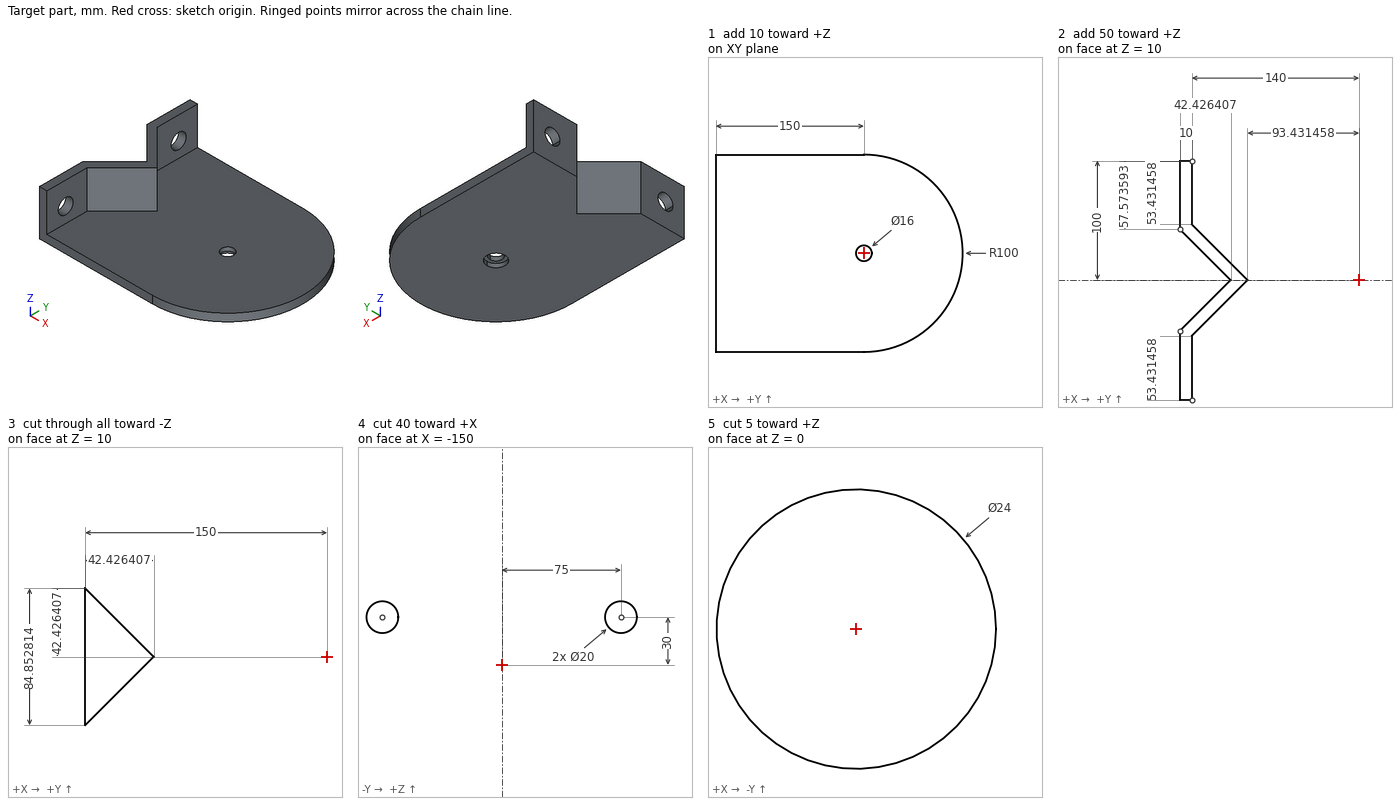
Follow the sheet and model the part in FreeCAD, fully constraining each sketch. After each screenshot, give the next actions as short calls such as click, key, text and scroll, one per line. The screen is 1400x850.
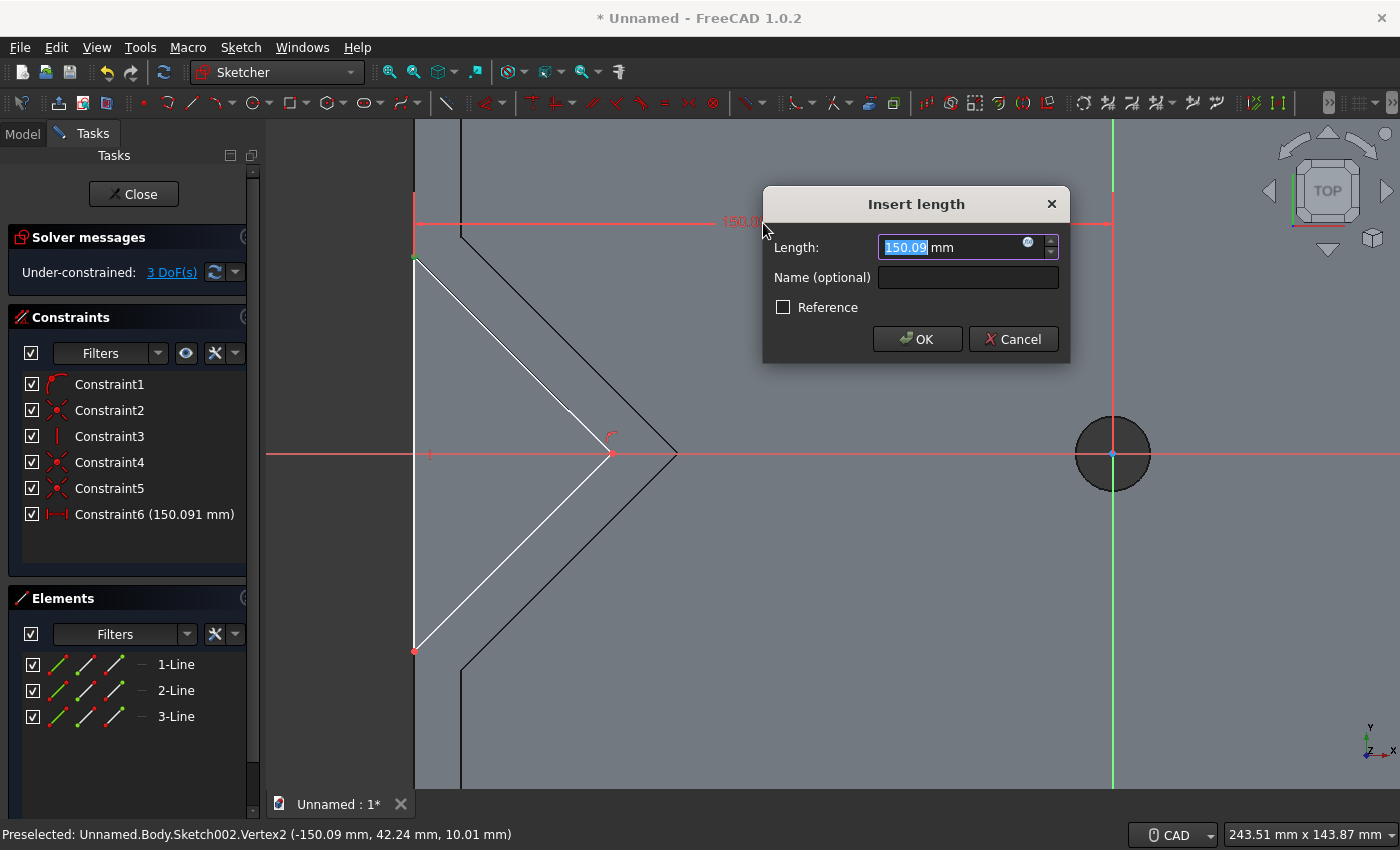
text(150)
key(Return)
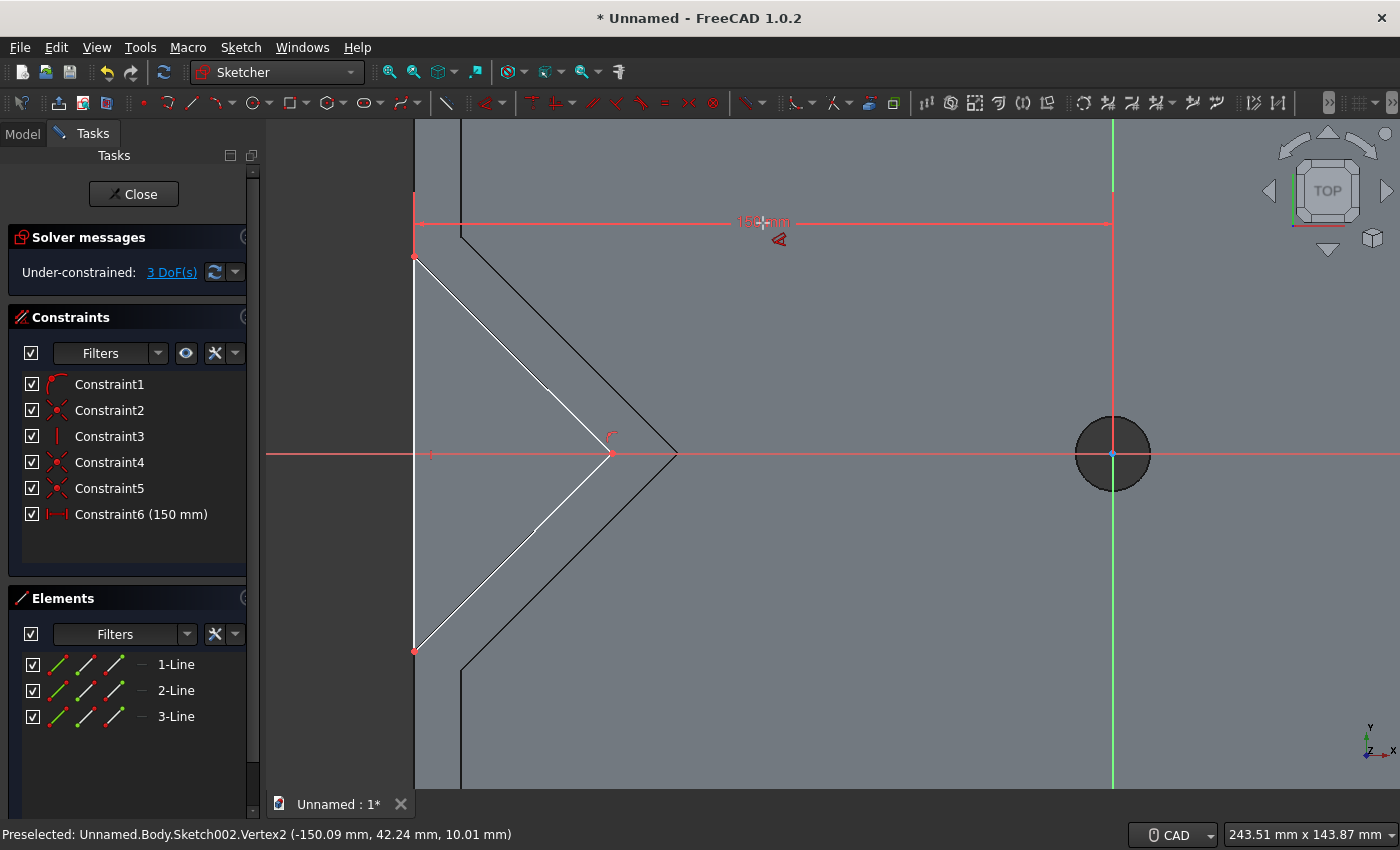
click(414, 376)
click(380, 364)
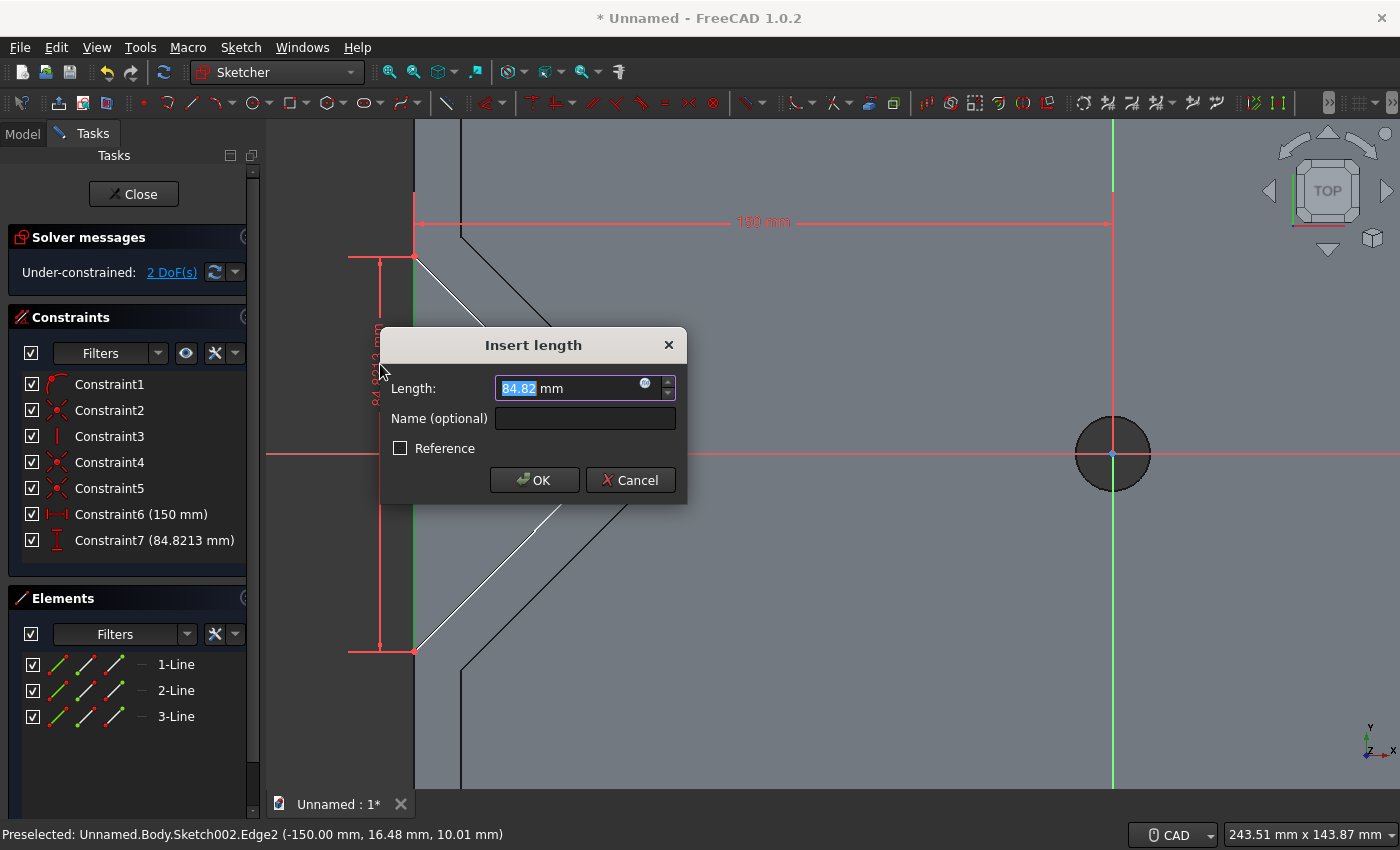
text(84.852814)
key(Return)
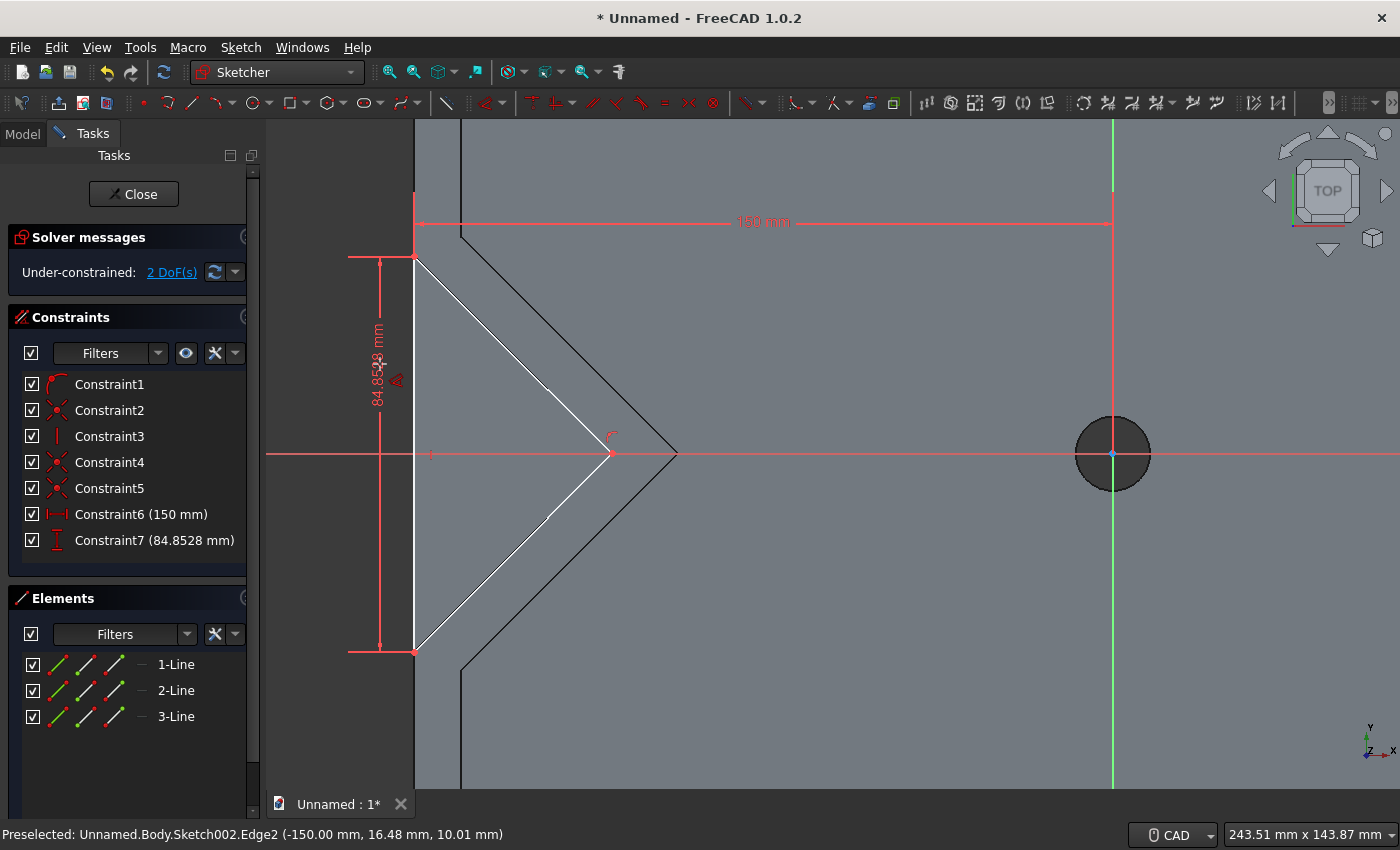
click(414, 257)
click(1147, 355)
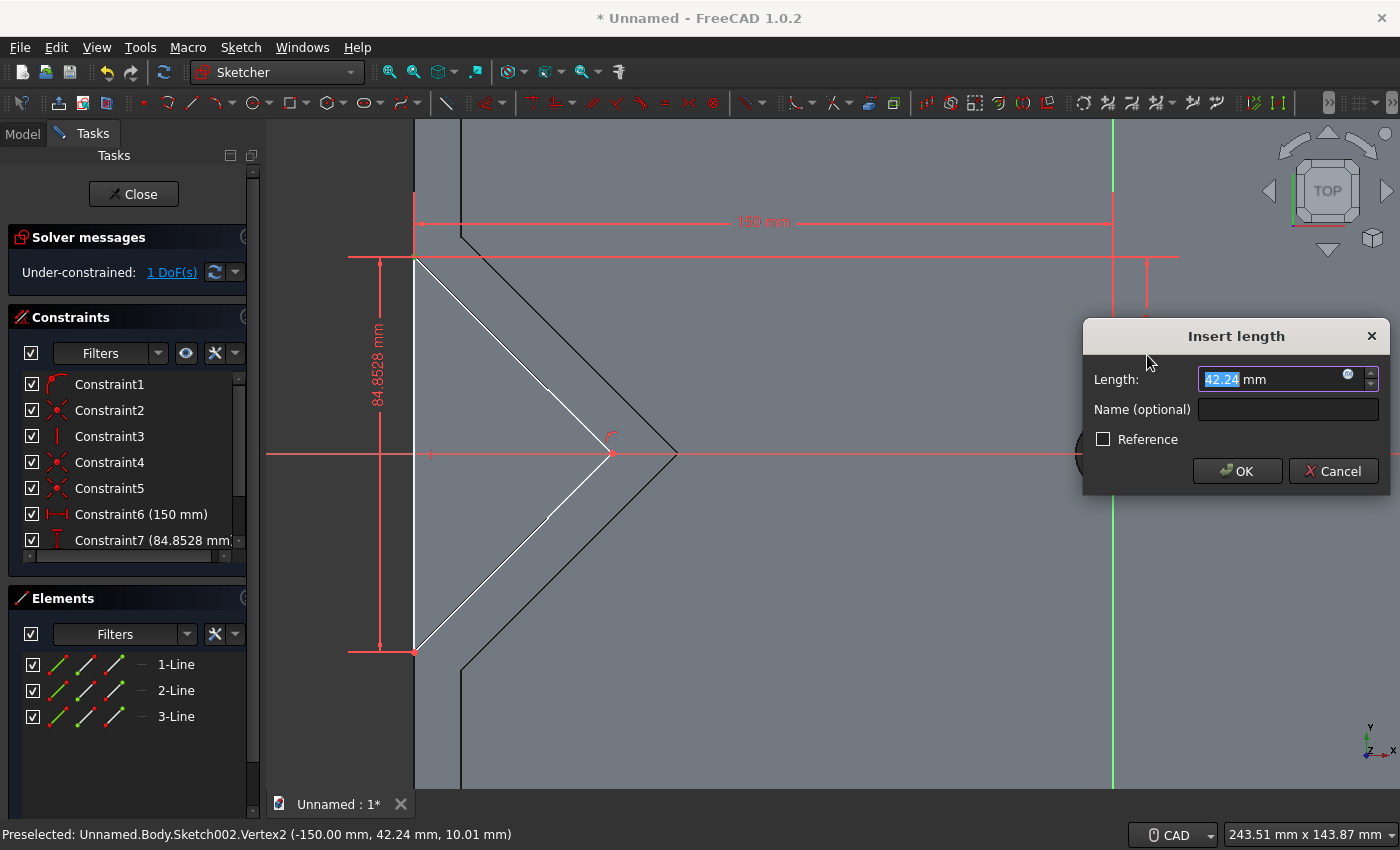
text(42.426407)
key(Return)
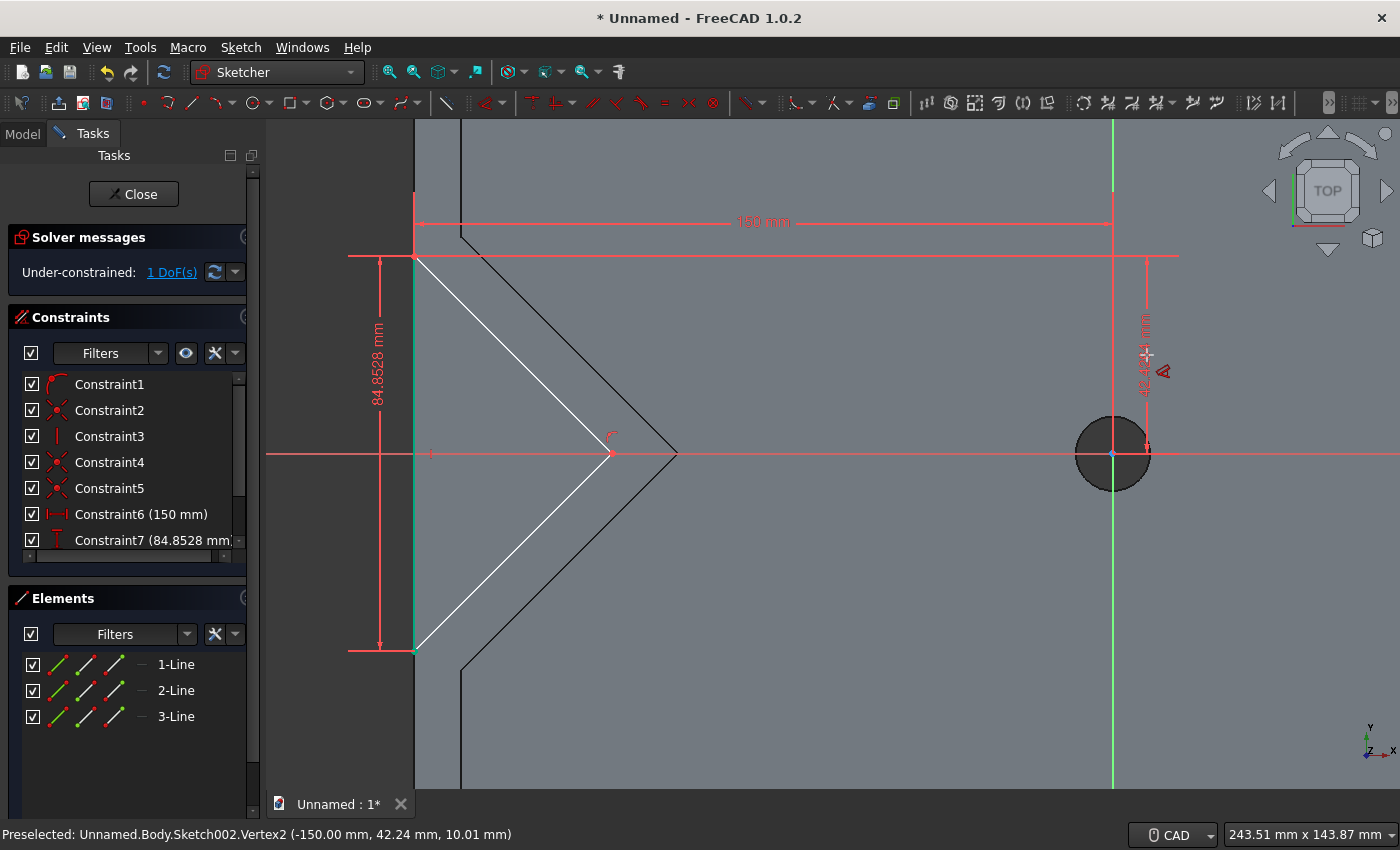
click(553, 394)
click(513, 222)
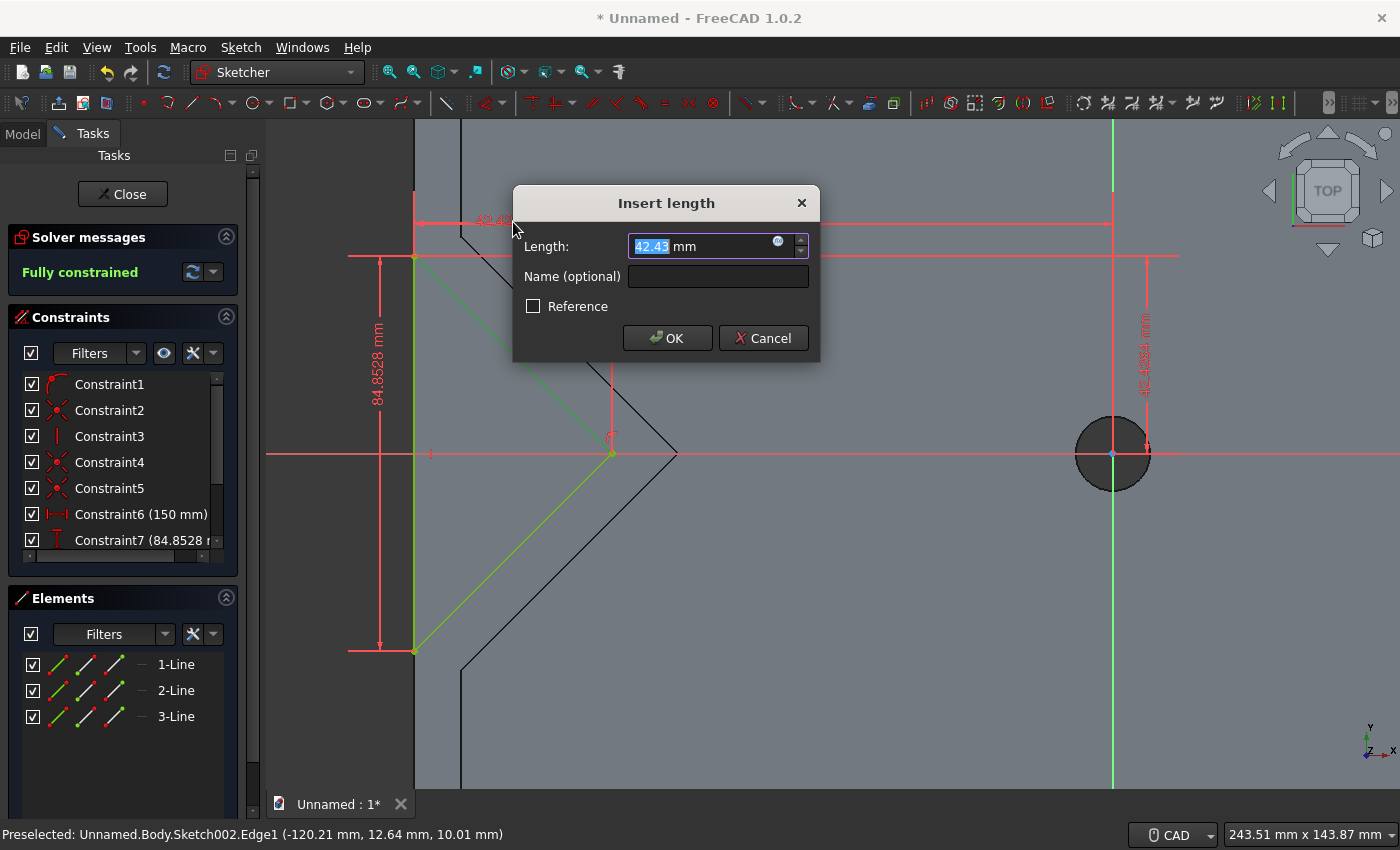
text(42.426407)
key(Return)
key(Escape)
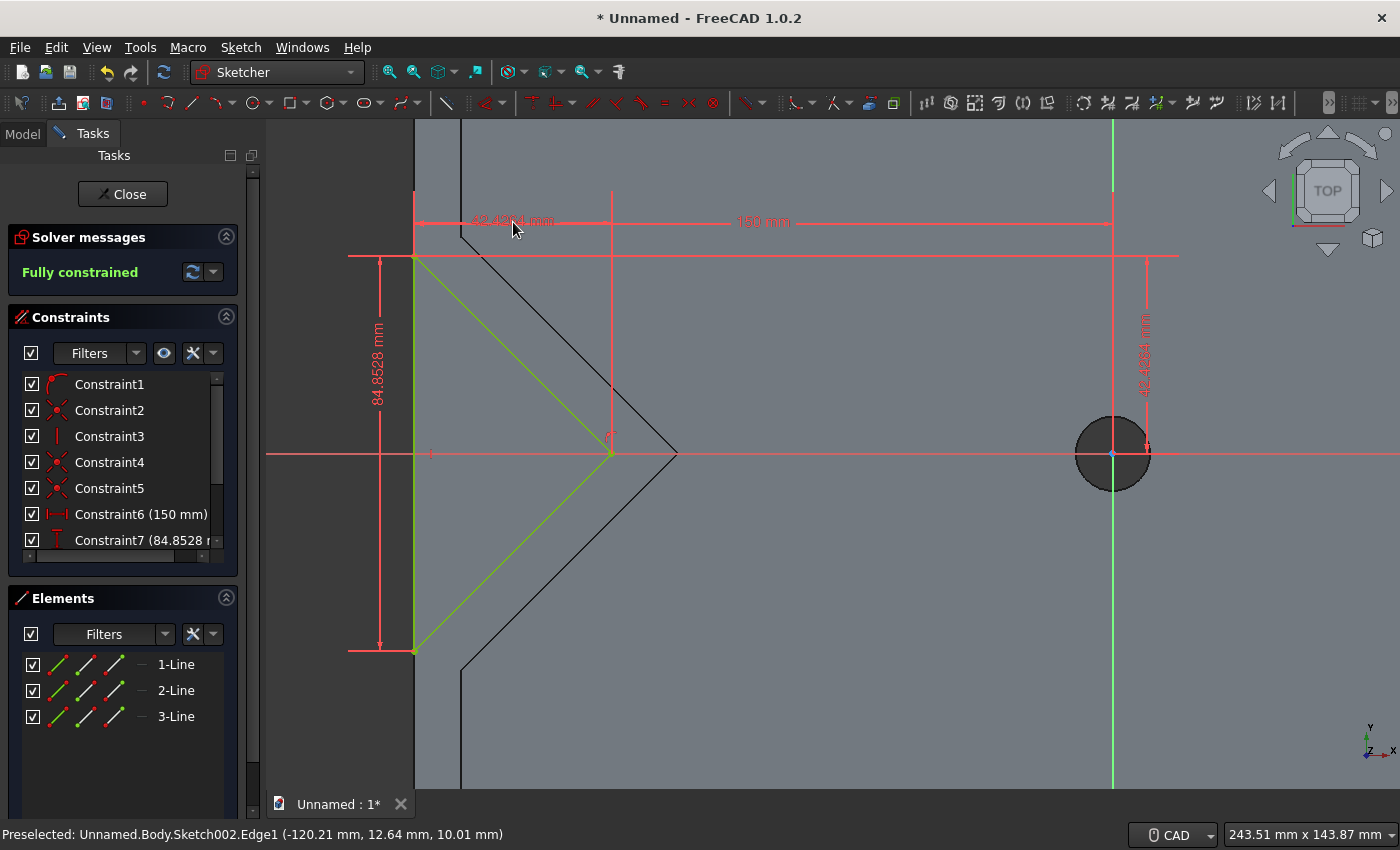
click(123, 194)